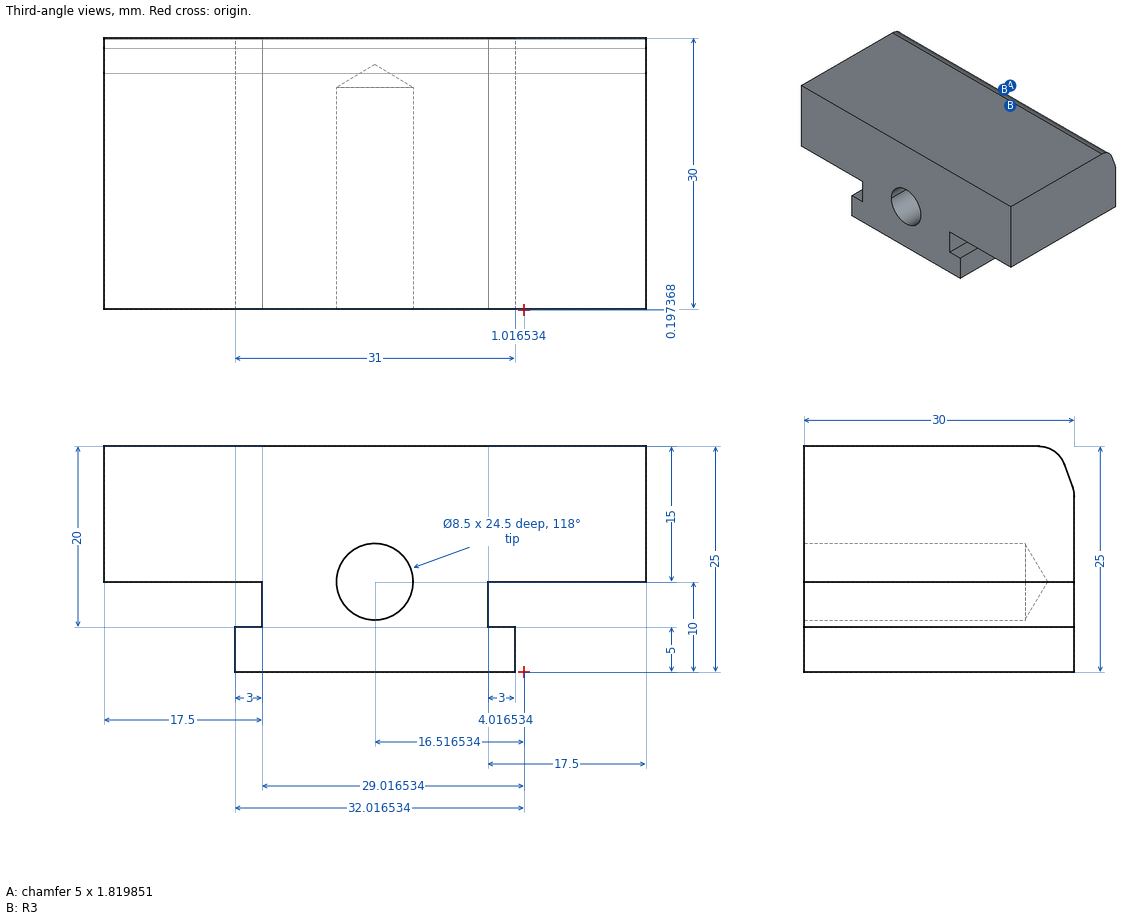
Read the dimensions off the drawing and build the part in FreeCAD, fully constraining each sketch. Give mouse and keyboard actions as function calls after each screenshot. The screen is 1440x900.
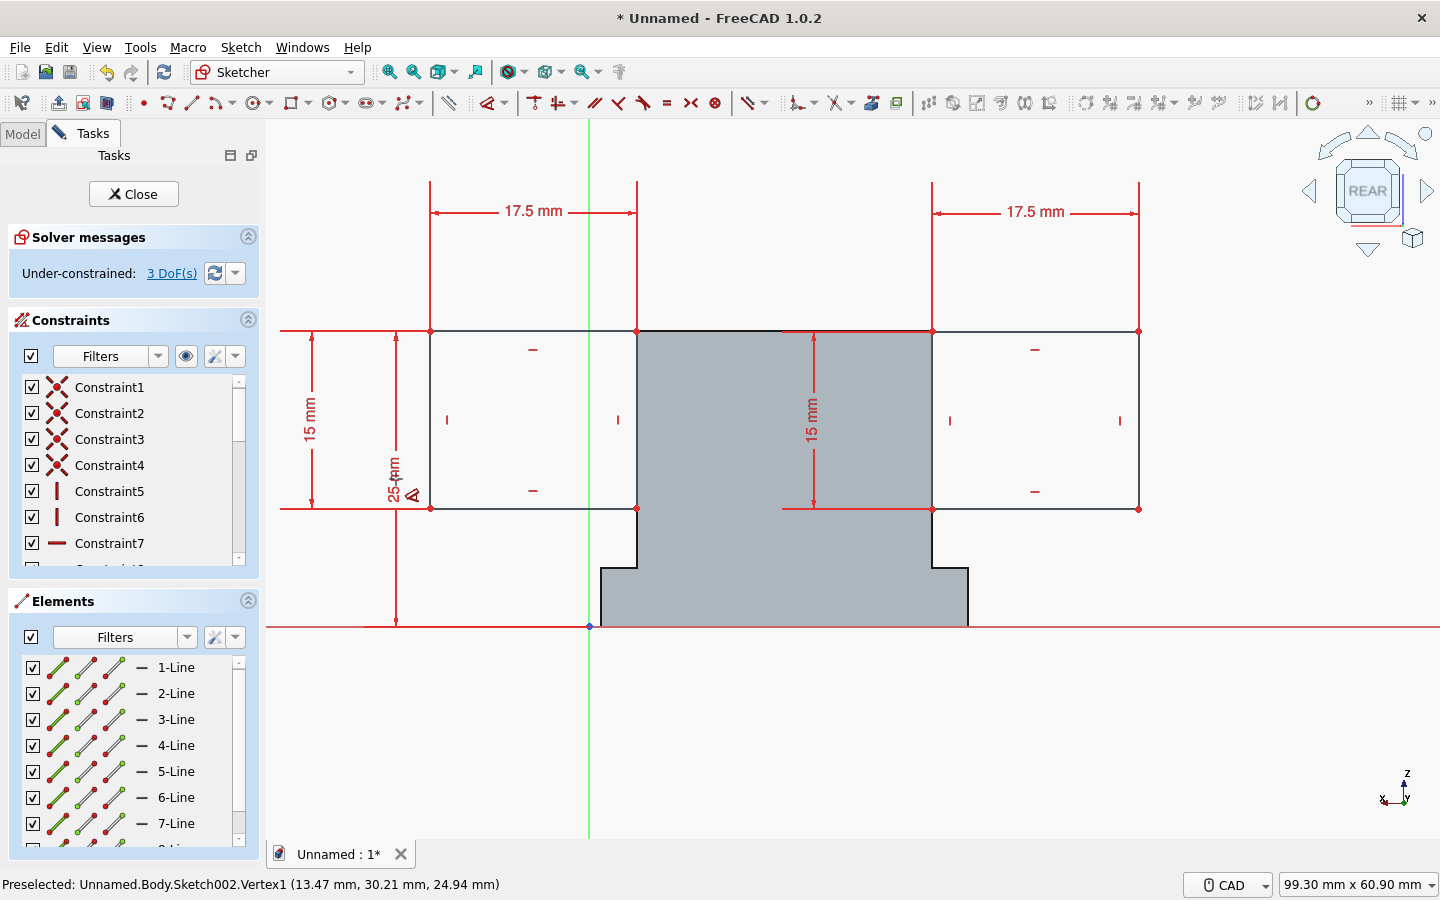
click(932, 332)
click(555, 479)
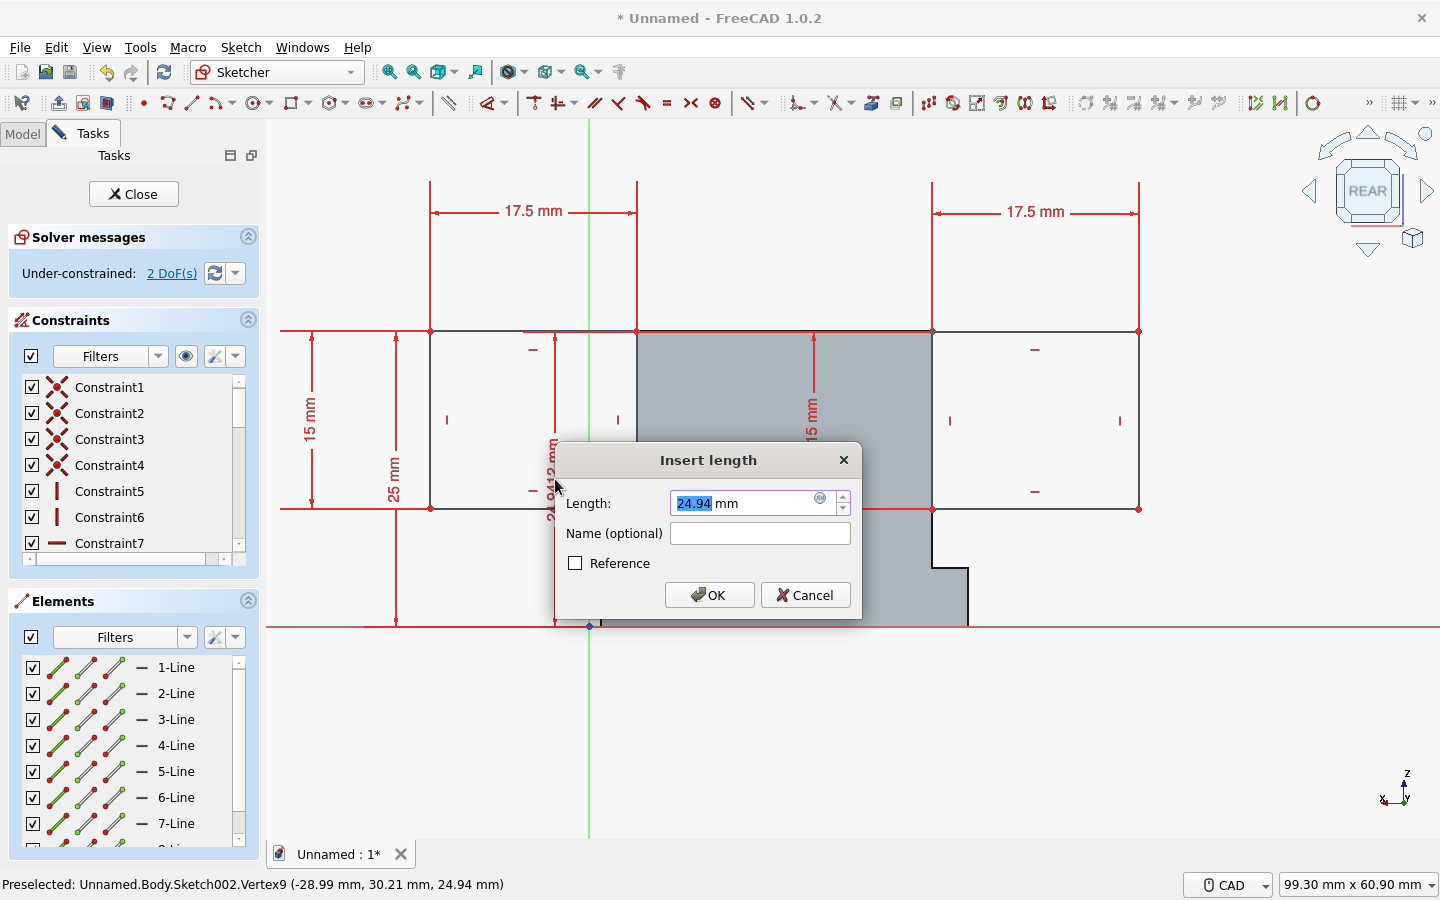
text(25)
key(Return)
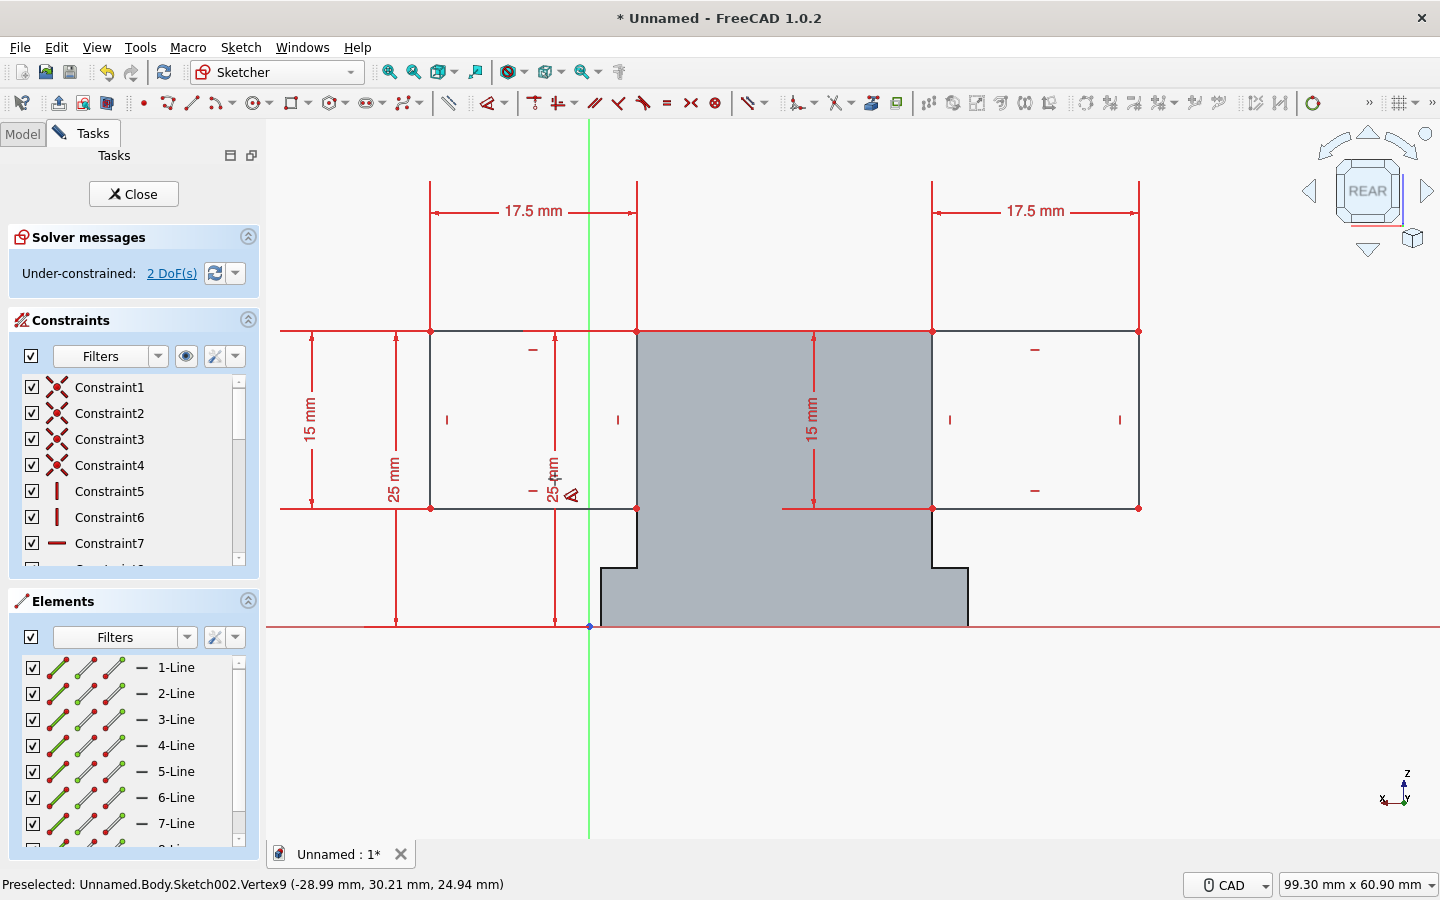
click(637, 509)
click(613, 661)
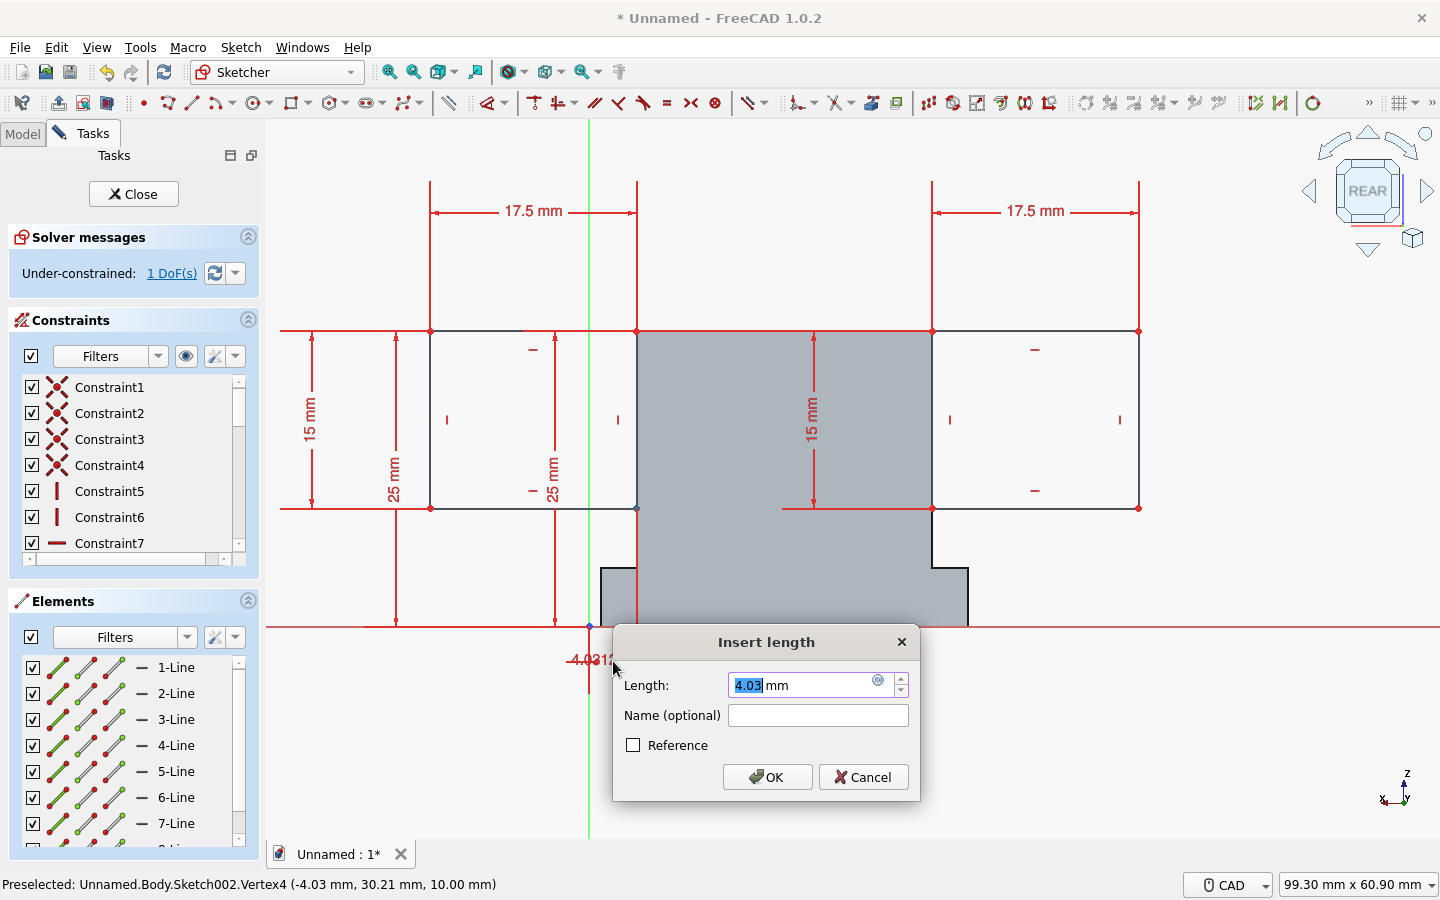
text(4.016534)
key(Return)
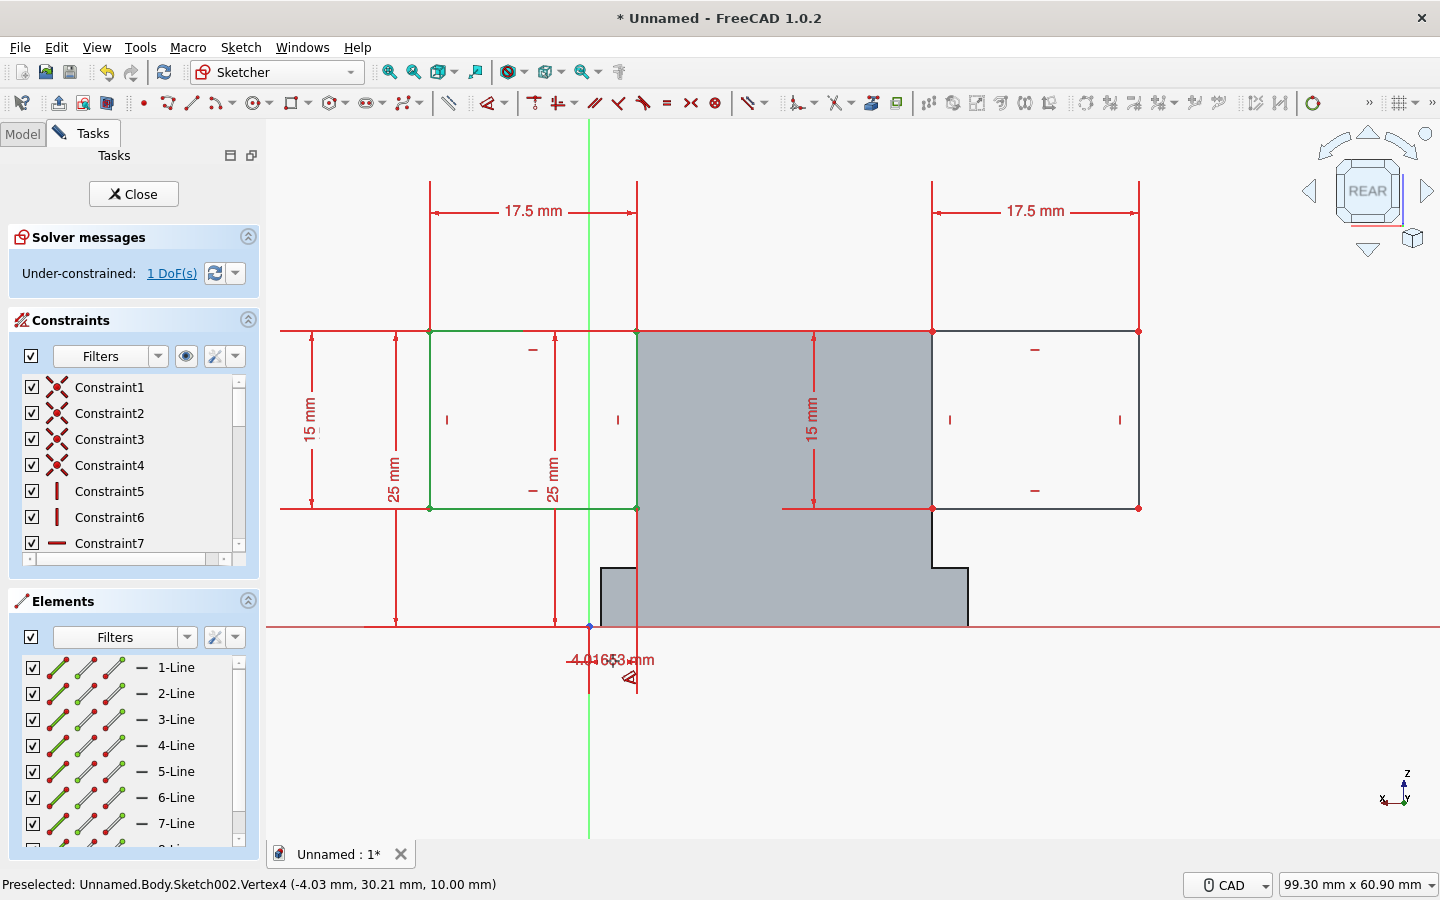
click(932, 331)
click(761, 661)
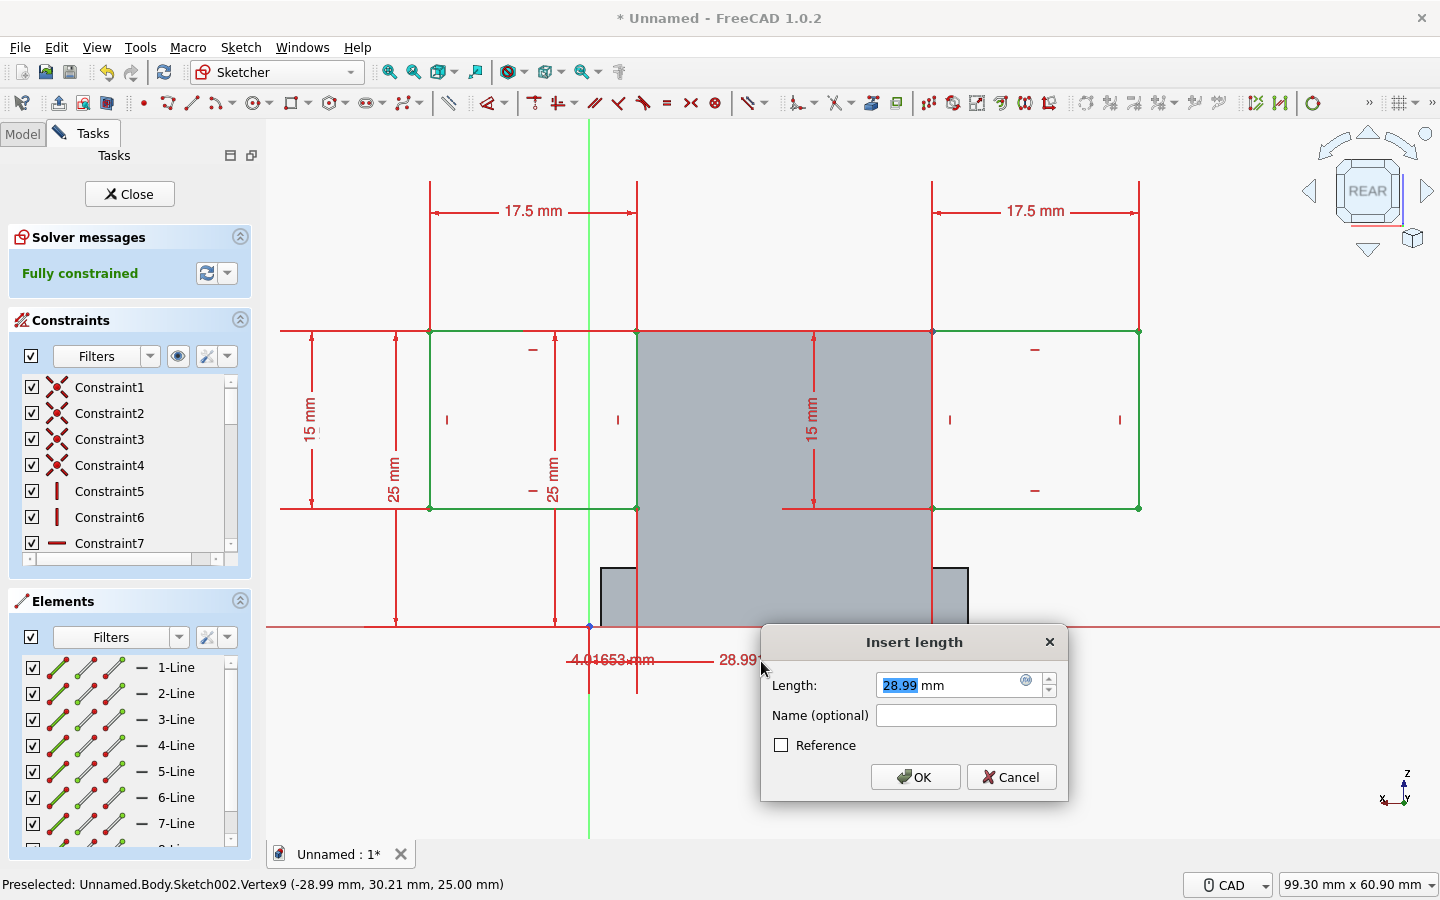
text(29.016534)
key(Return)
key(Escape)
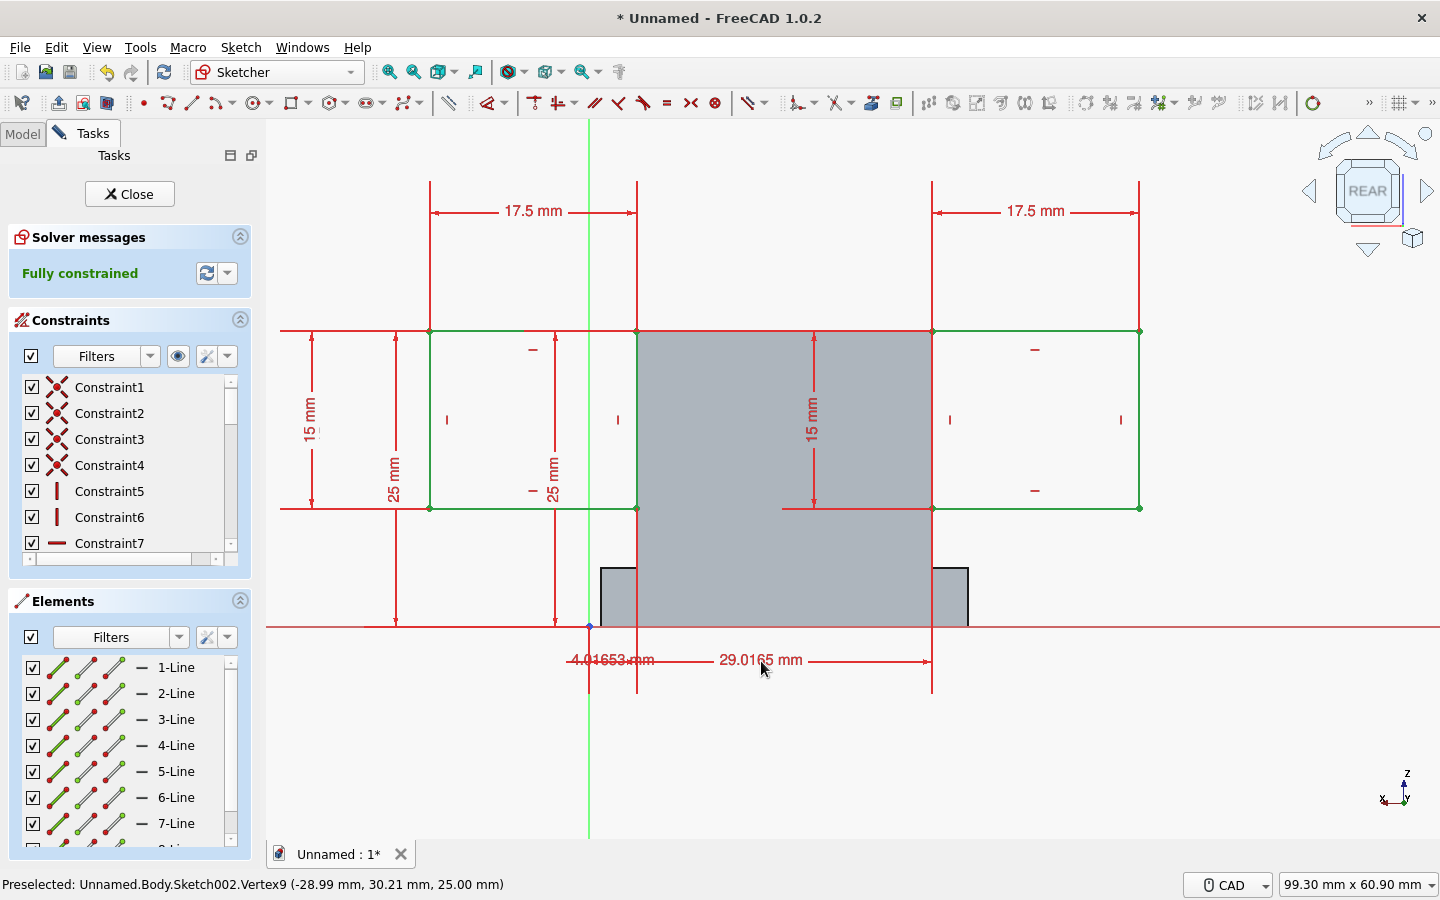
click(130, 194)